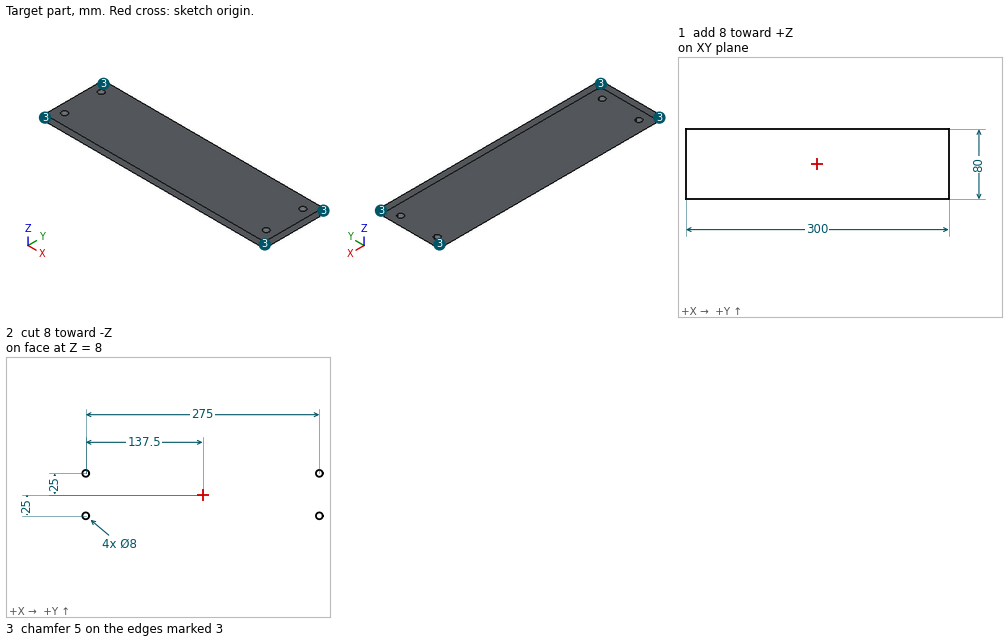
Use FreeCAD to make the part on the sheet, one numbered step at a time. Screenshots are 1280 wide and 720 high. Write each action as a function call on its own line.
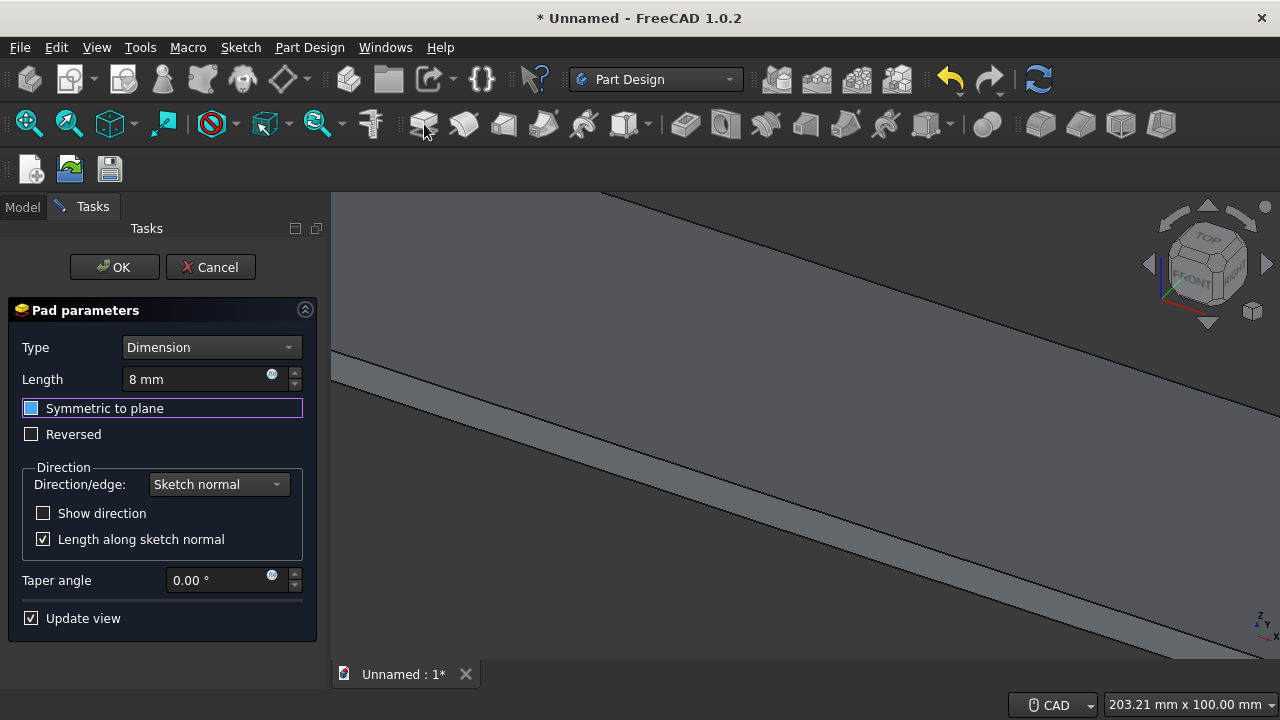
click(115, 267)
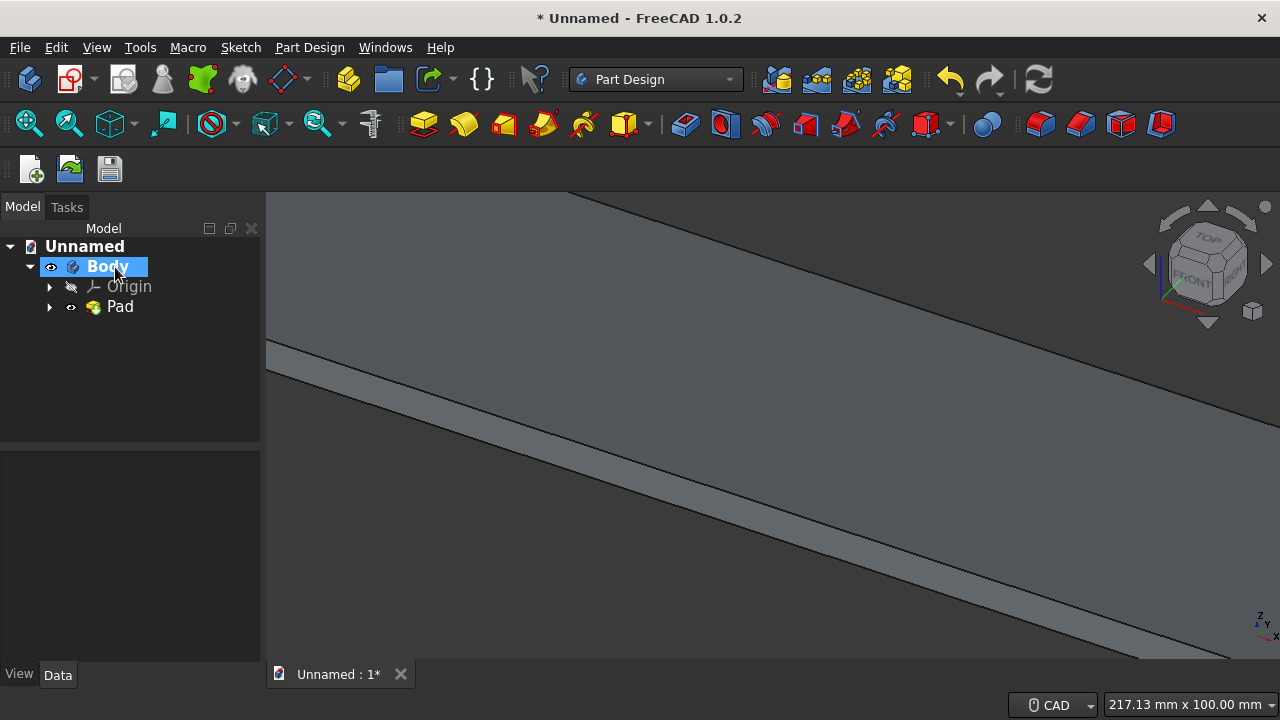
key(v)
key(f)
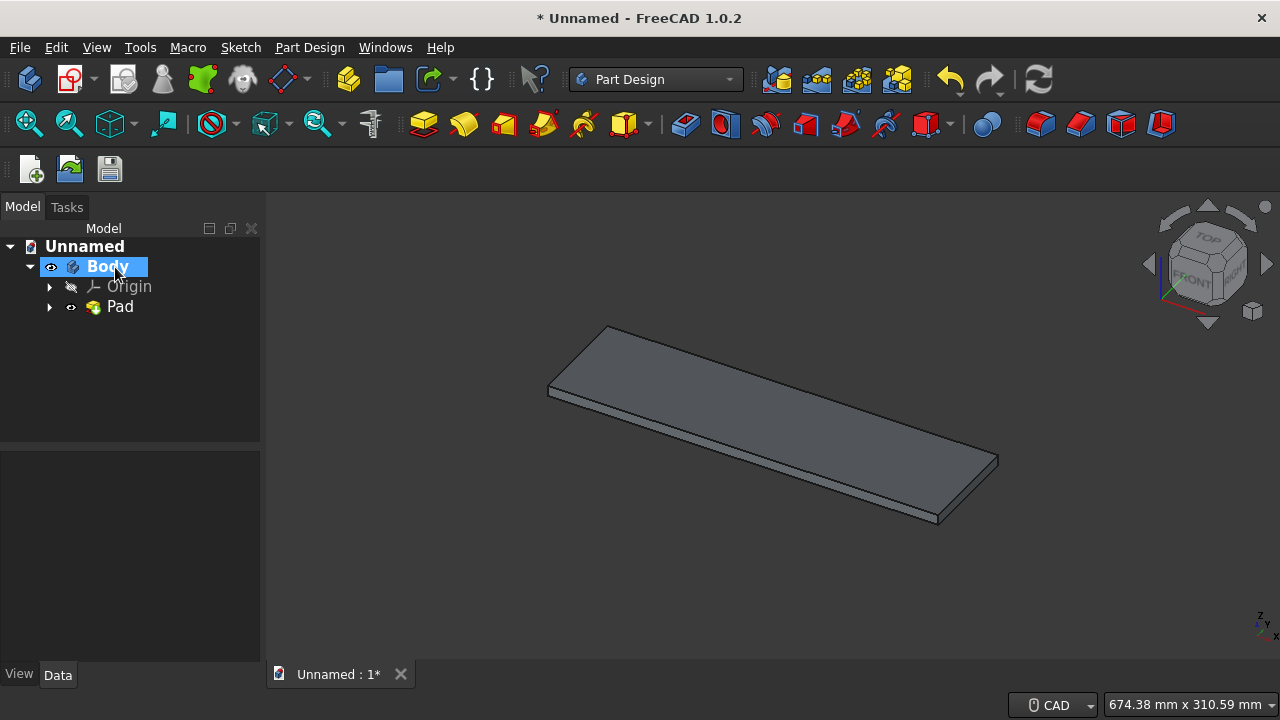
click(885, 457)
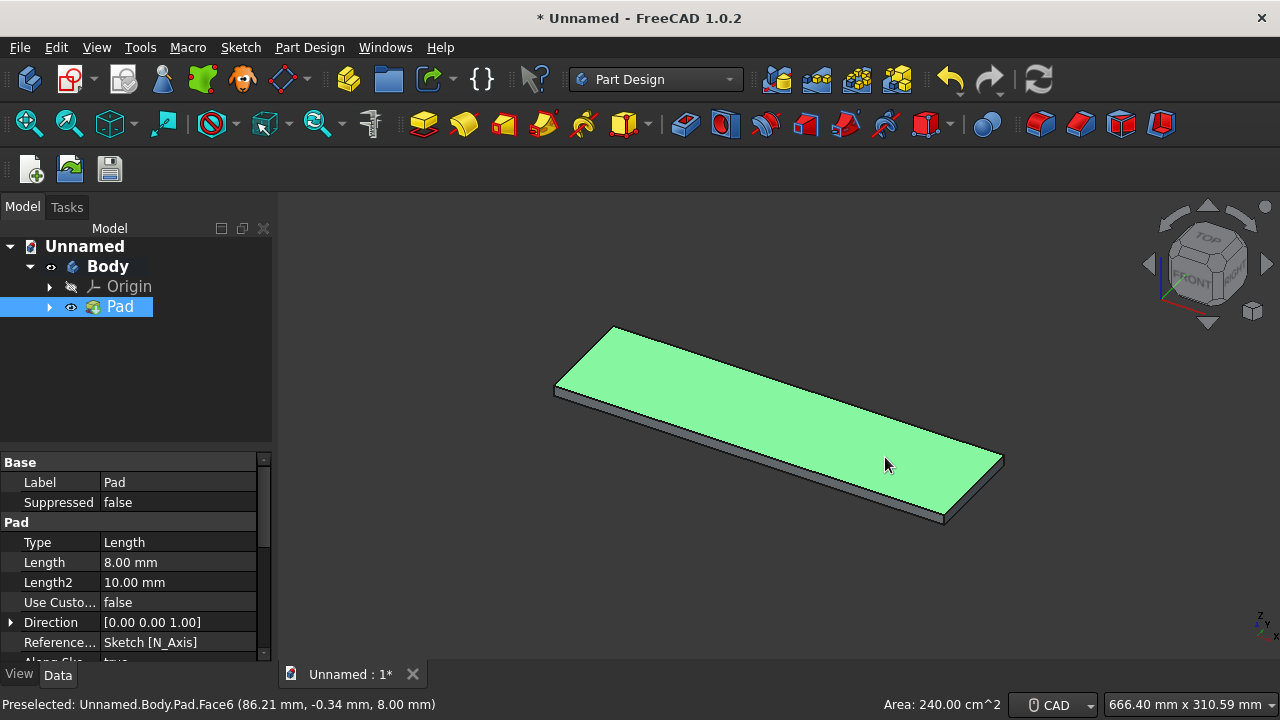
click(70, 80)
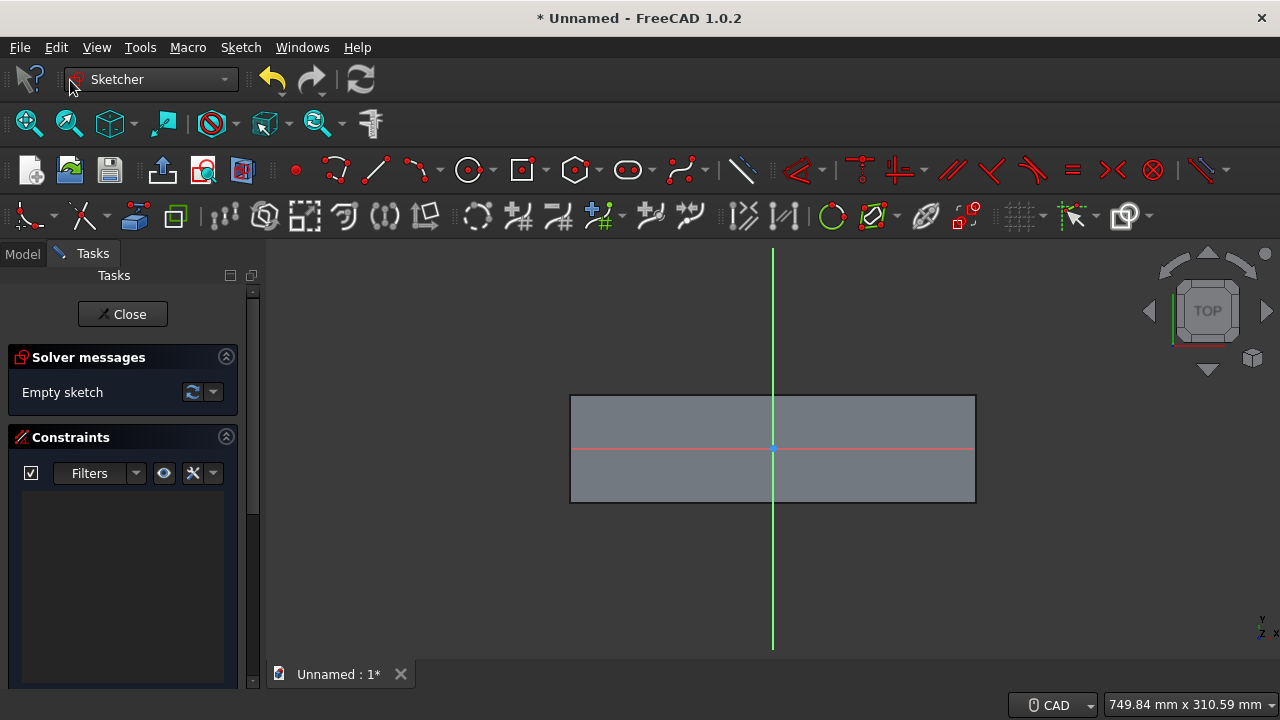
scroll(912, 449, up, 2)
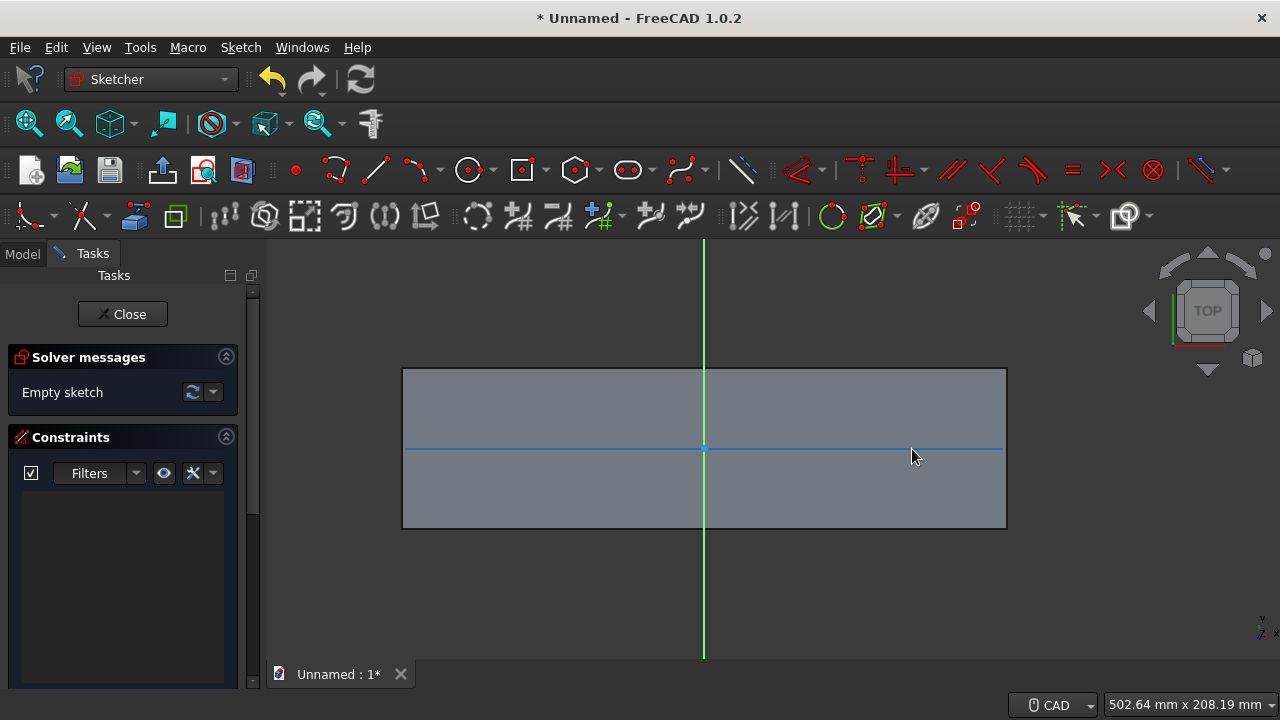
key(g)
key(c)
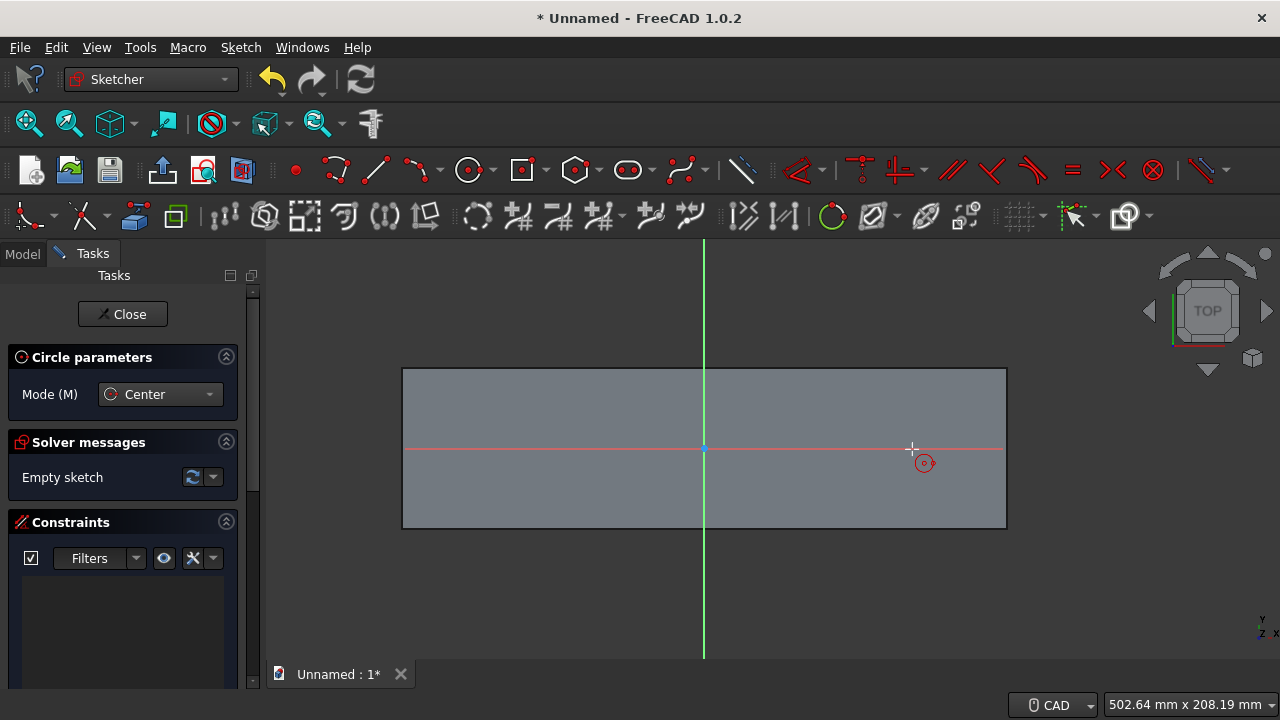
scroll(427, 398, up, 6)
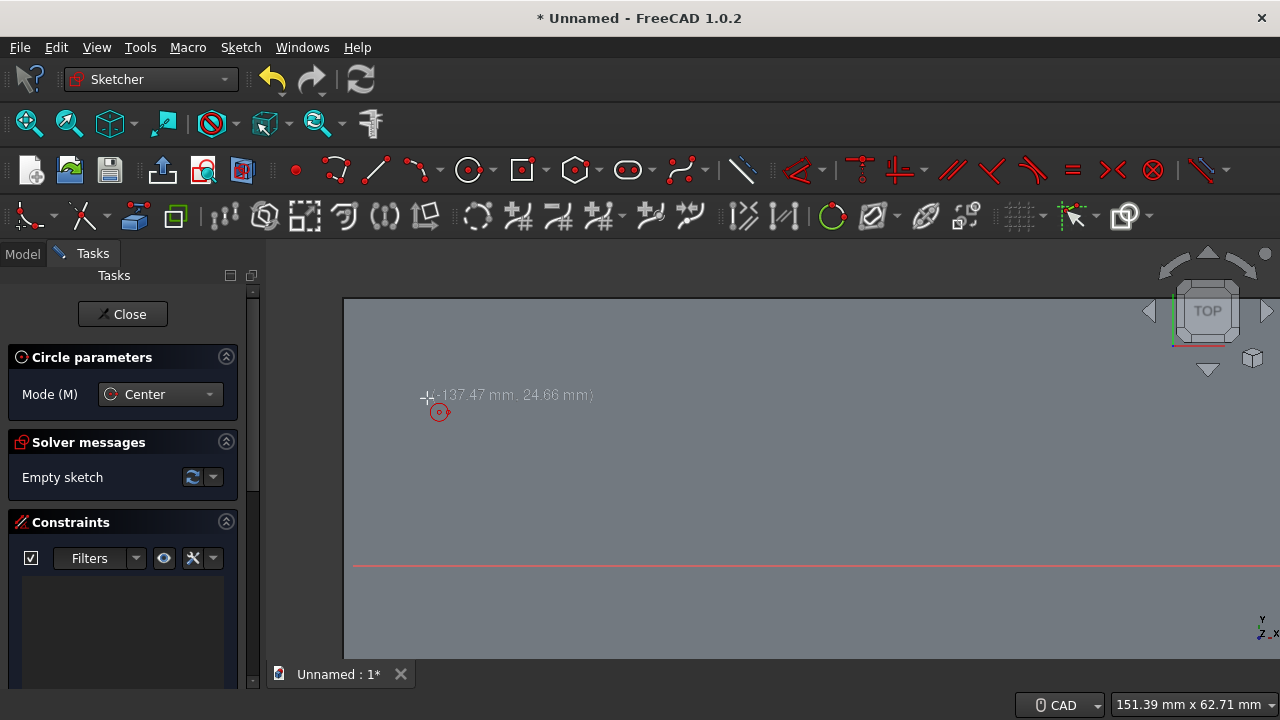
click(426, 398)
move(445, 379)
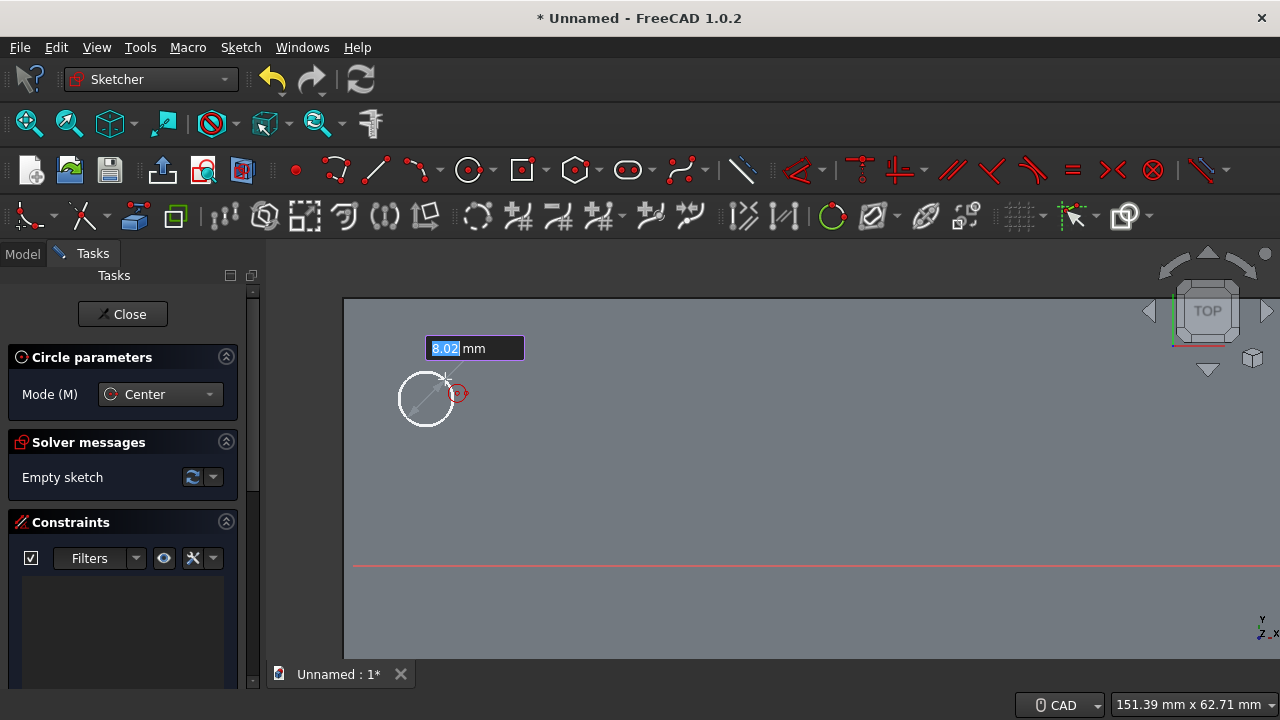
text(8)
key(Return)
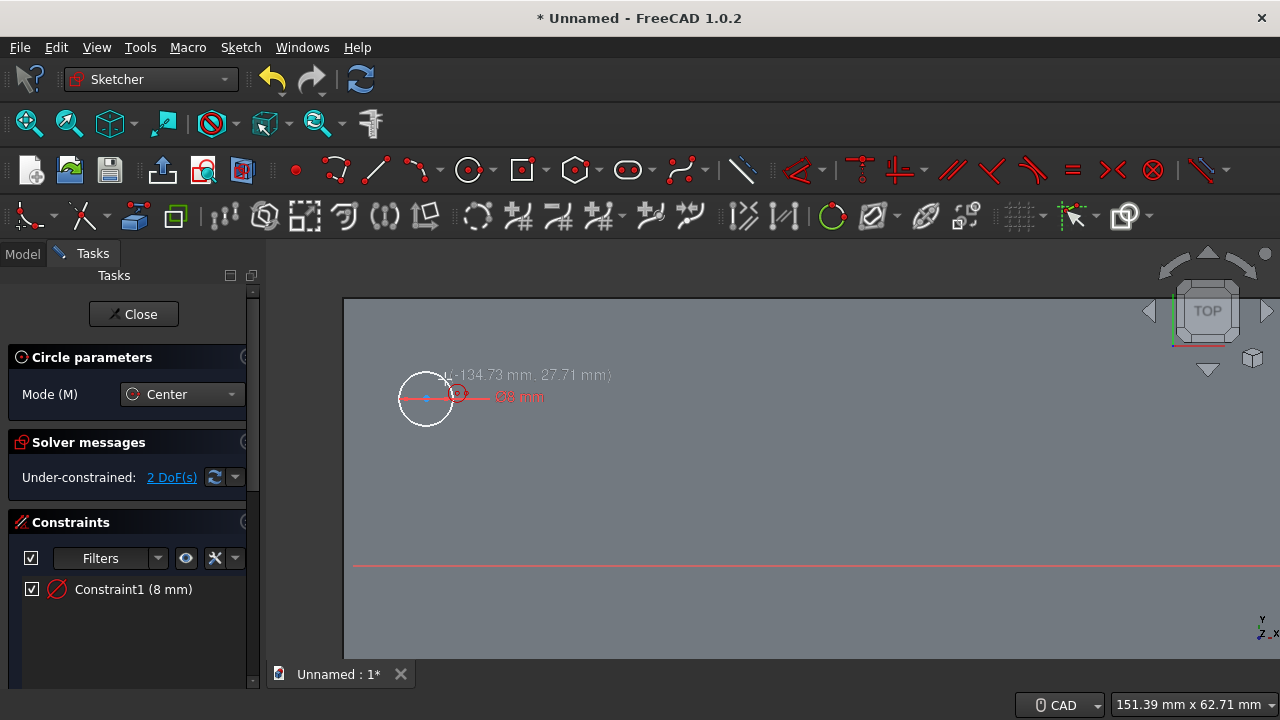
scroll(427, 399, down, 6)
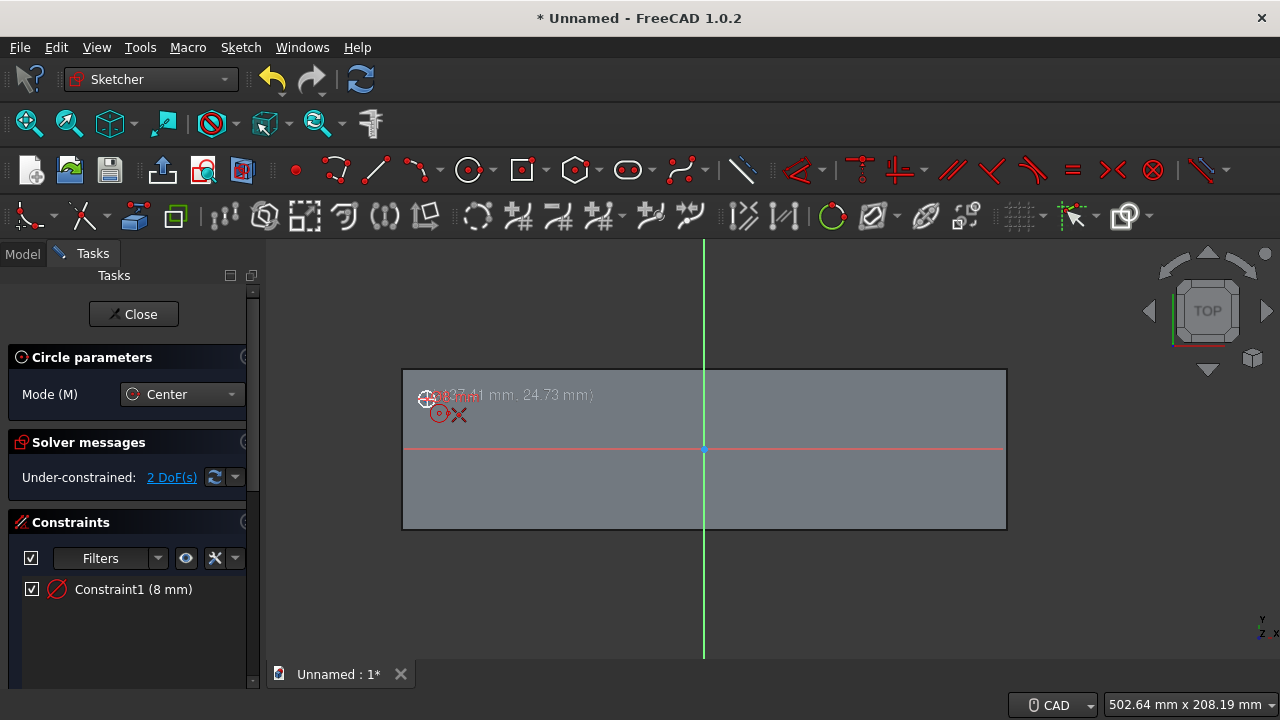
scroll(427, 500, up, 6)